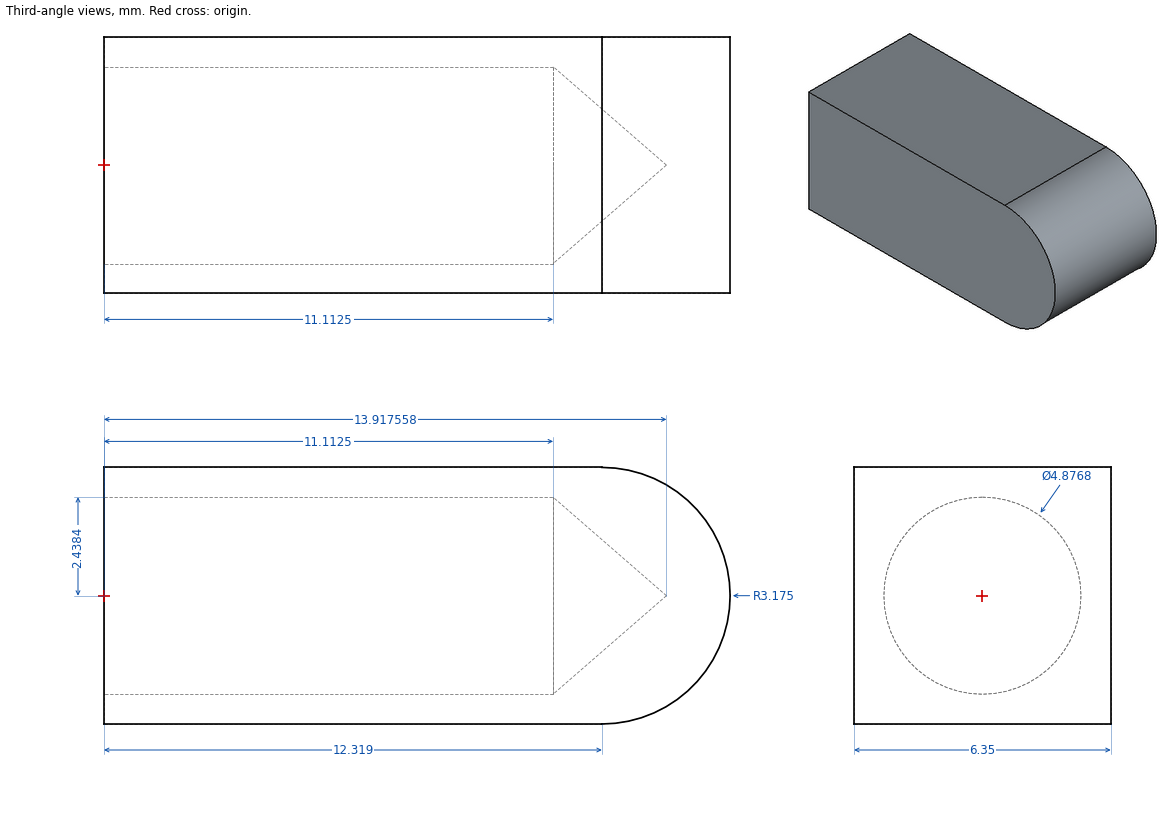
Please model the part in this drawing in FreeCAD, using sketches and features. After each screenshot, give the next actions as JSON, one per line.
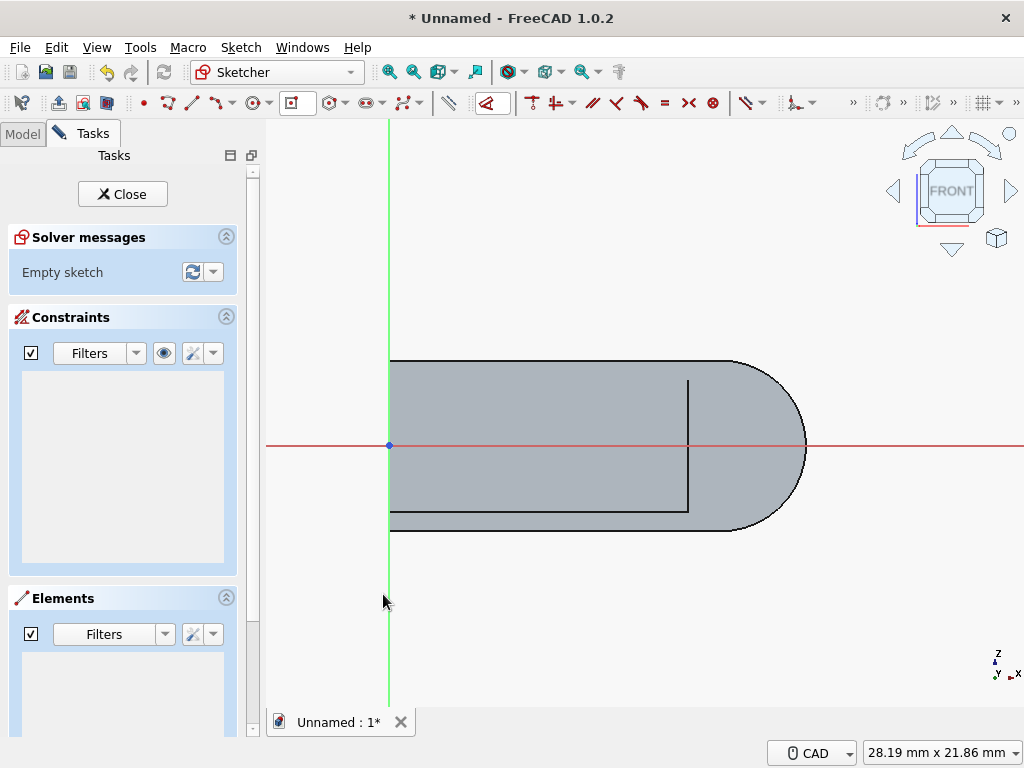
{"action": "key", "text": "g m"}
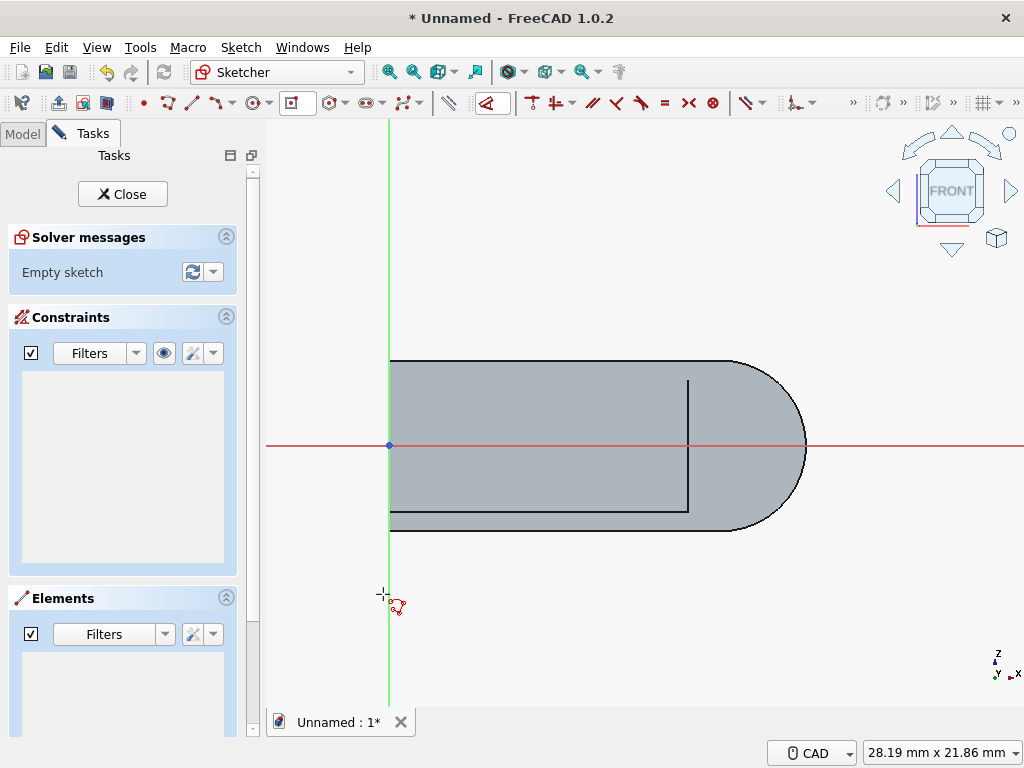
{"action": "left_click", "coordinate": [389, 446]}
{"action": "left_click", "coordinate": [398, 380]}
{"action": "left_click", "coordinate": [688, 380]}
{"action": "left_click", "coordinate": [764, 437]}
{"action": "left_click", "coordinate": [389, 446]}
{"action": "key", "text": "Escape"}
{"action": "key", "text": "Escape"}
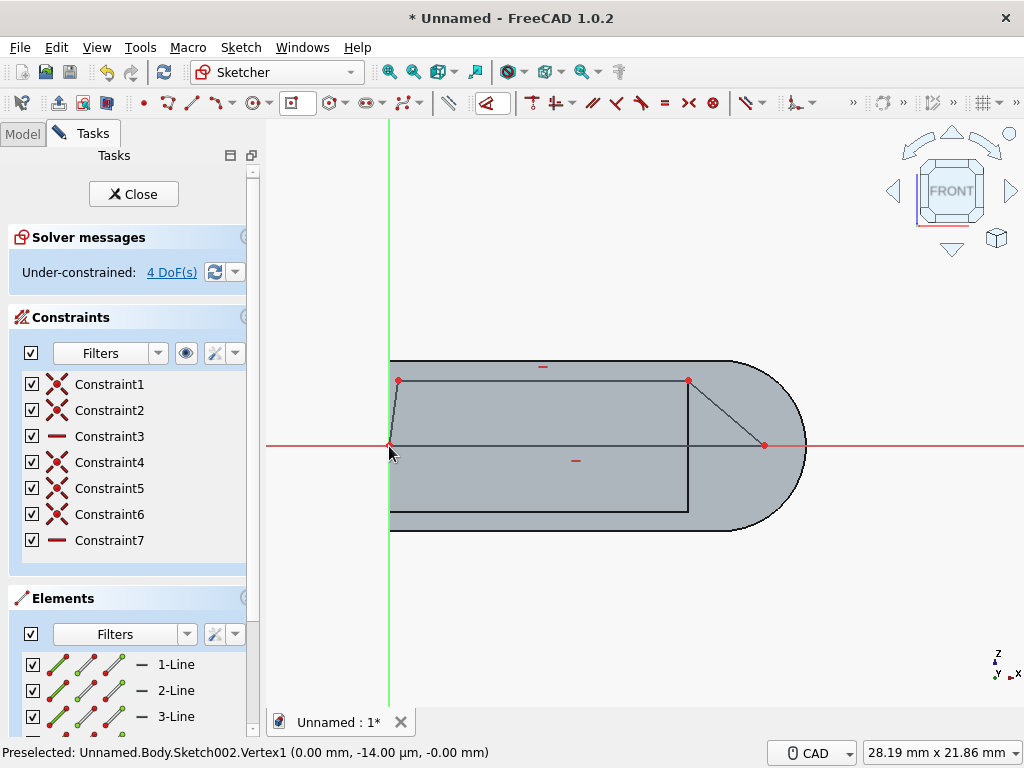
{"action": "left_click", "coordinate": [392, 426]}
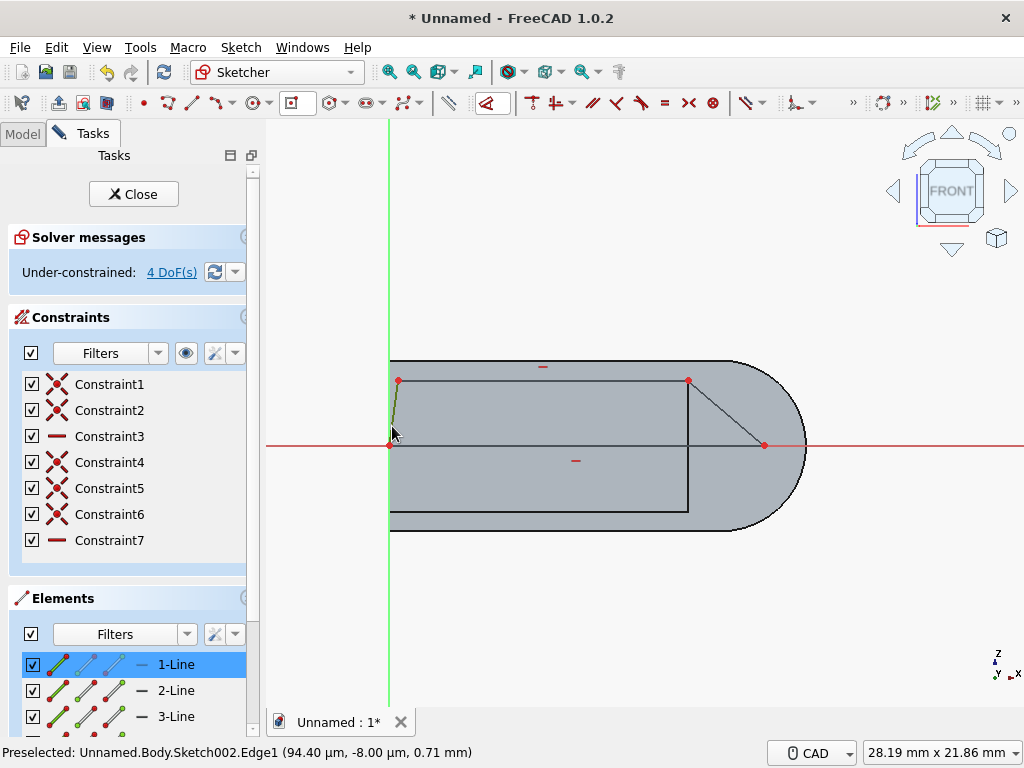
{"action": "key", "text": "v"}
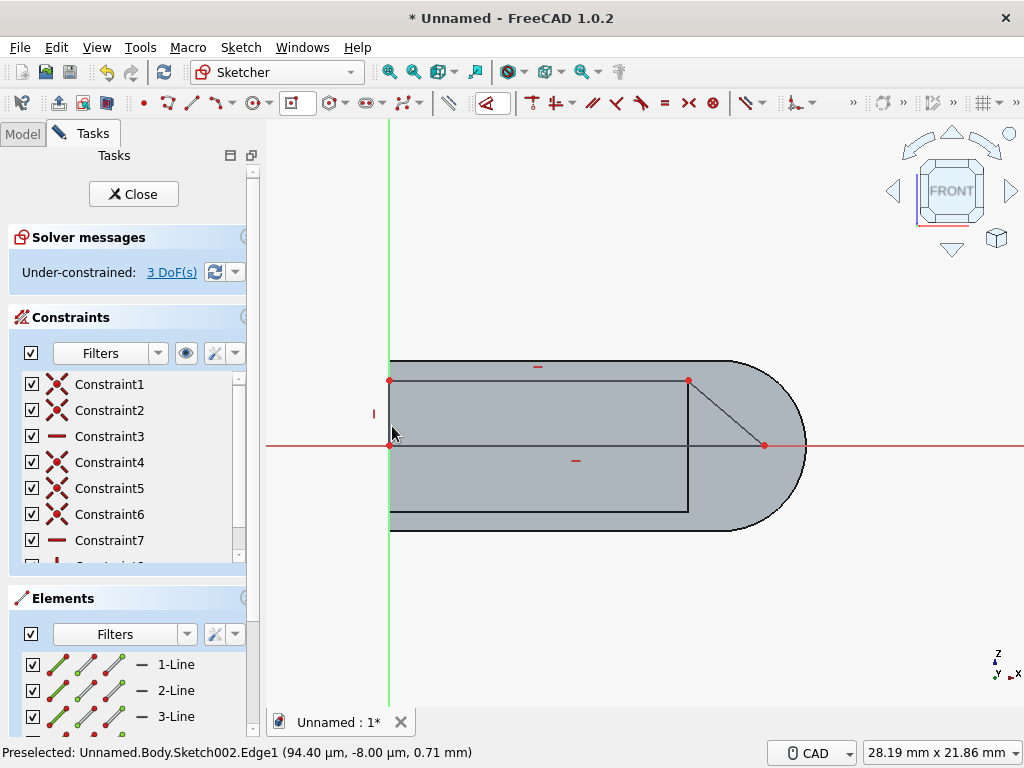
{"action": "left_click", "coordinate": [486, 104]}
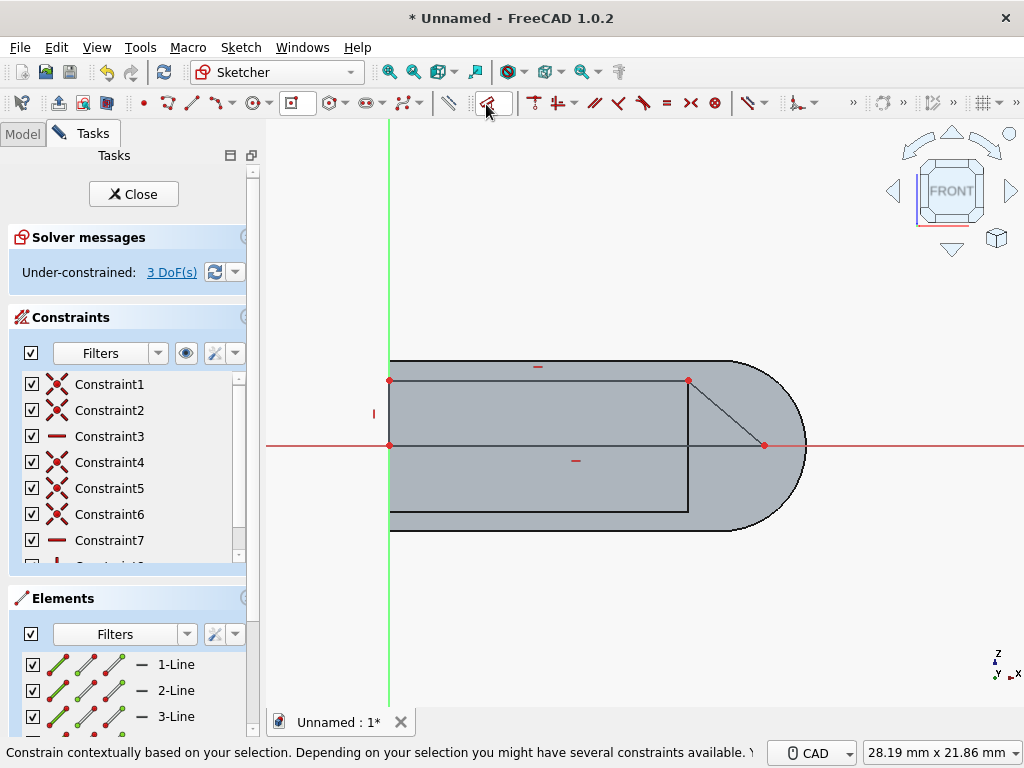
{"action": "left_click", "coordinate": [389, 426]}
{"action": "left_click", "coordinate": [355, 413]}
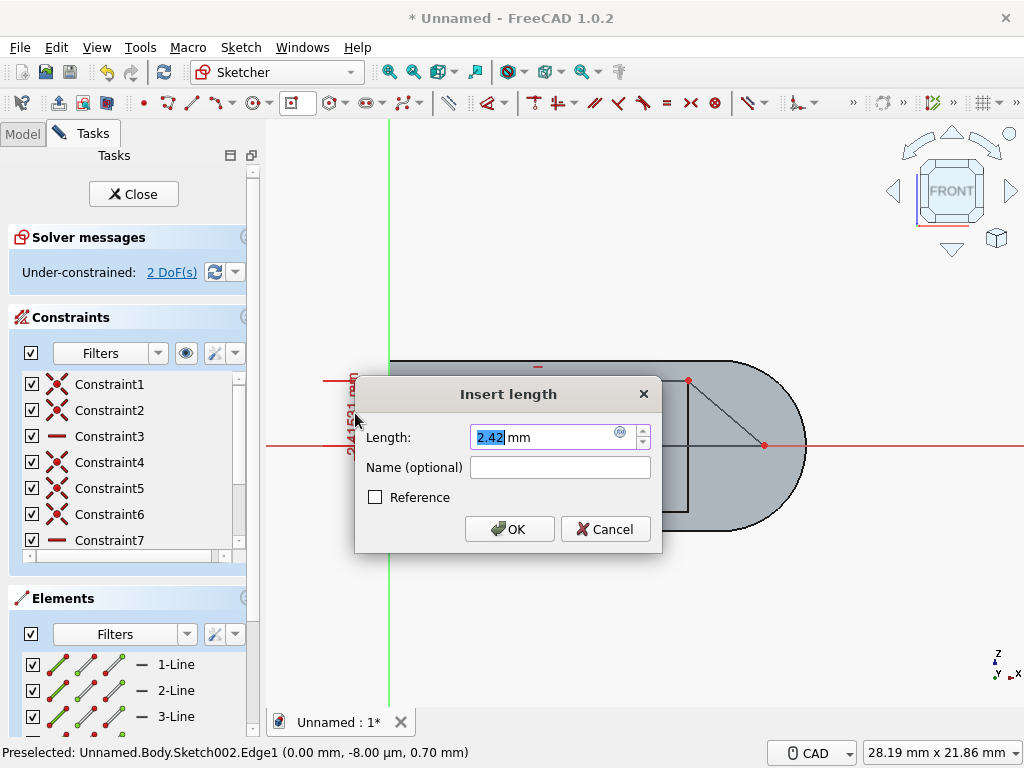
{"action": "type", "text": "2.4384"}
{"action": "key", "text": "Return"}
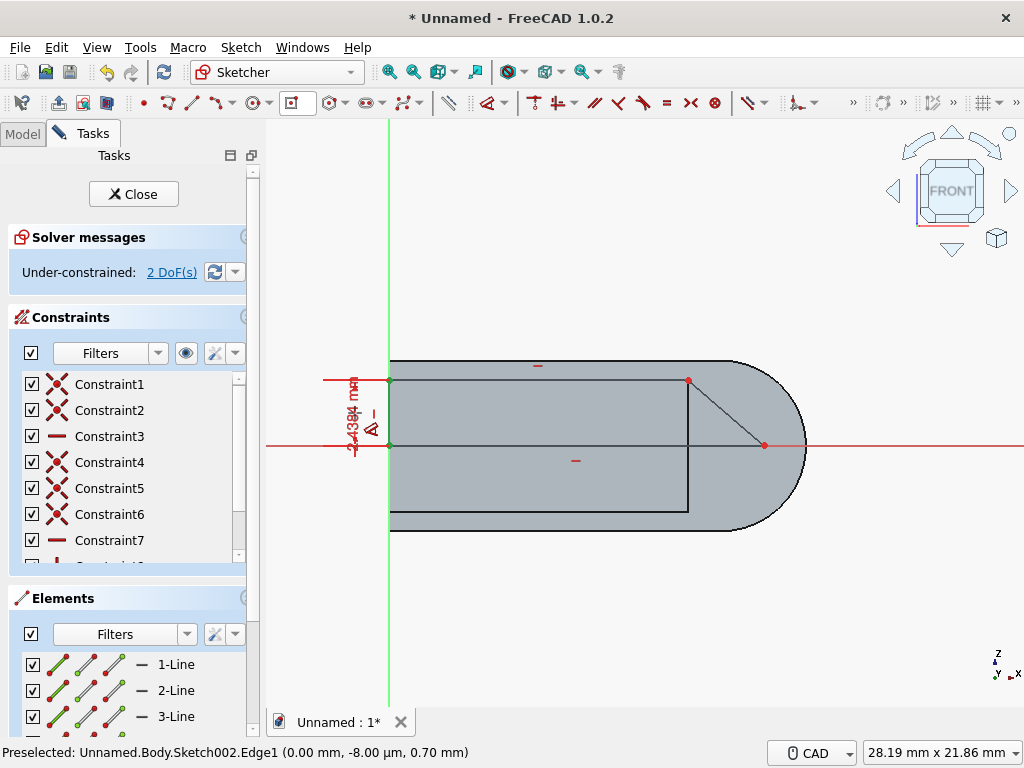
{"action": "left_click", "coordinate": [479, 380]}
{"action": "left_click", "coordinate": [539, 346]}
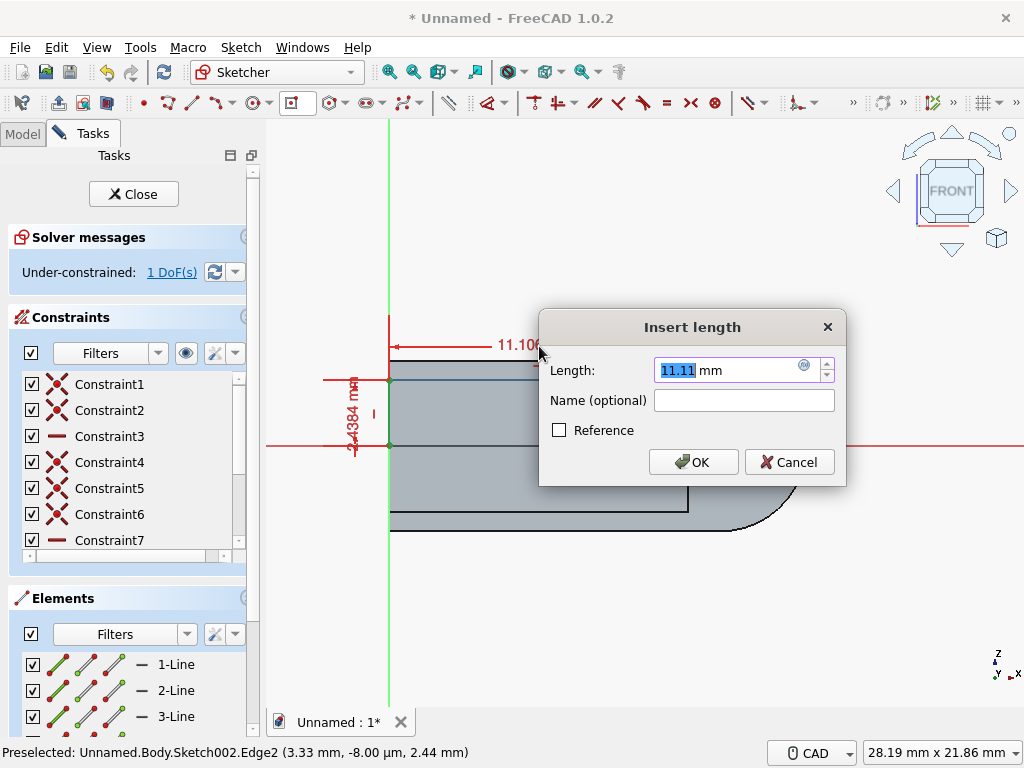
{"action": "type", "text": "11.1125"}
{"action": "key", "text": "Return"}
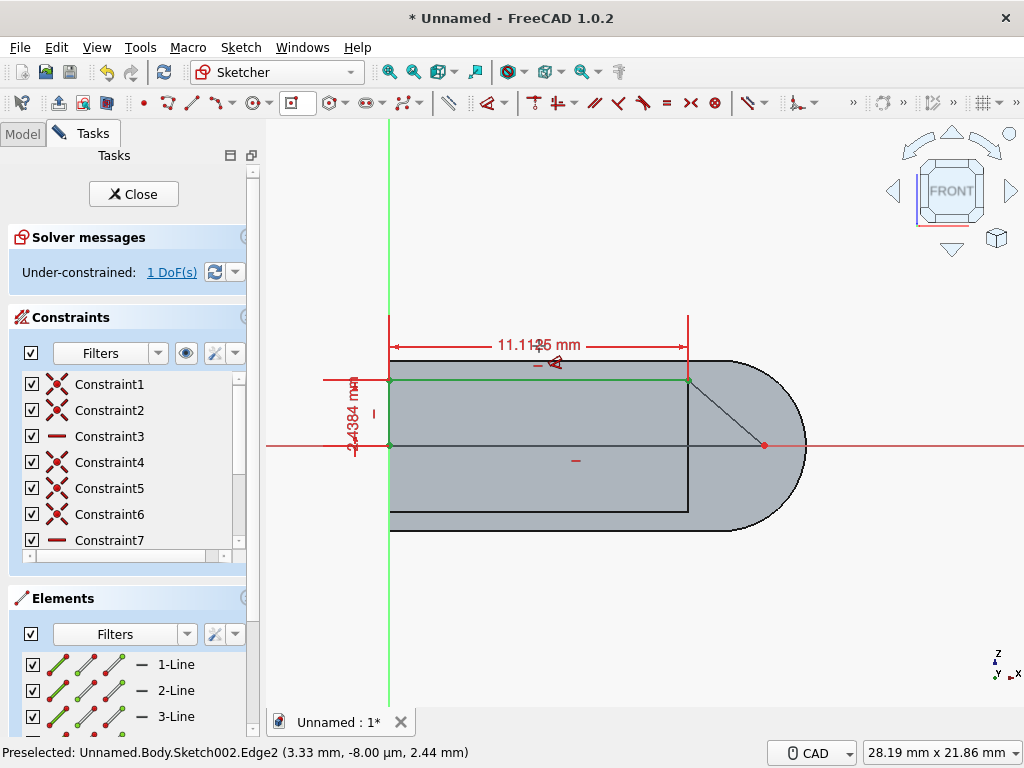
{"action": "left_click", "coordinate": [652, 446]}
{"action": "left_click", "coordinate": [577, 480]}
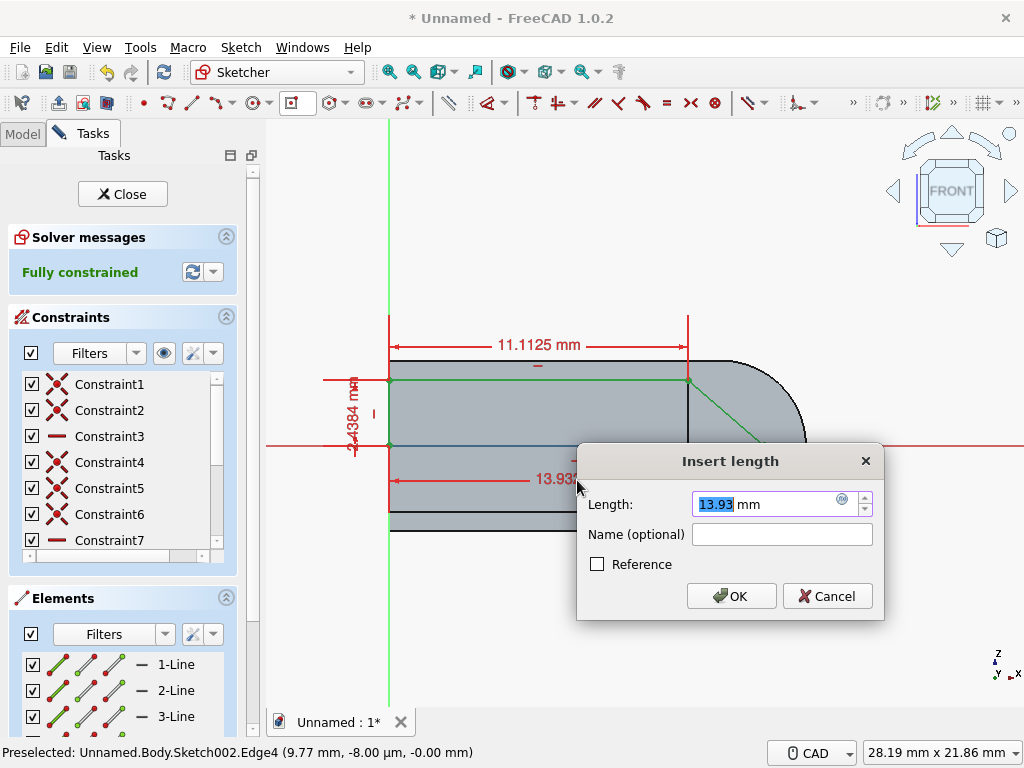
{"action": "type", "text": "13.917558"}
{"action": "key", "text": "Return"}
{"action": "key", "text": "Escape"}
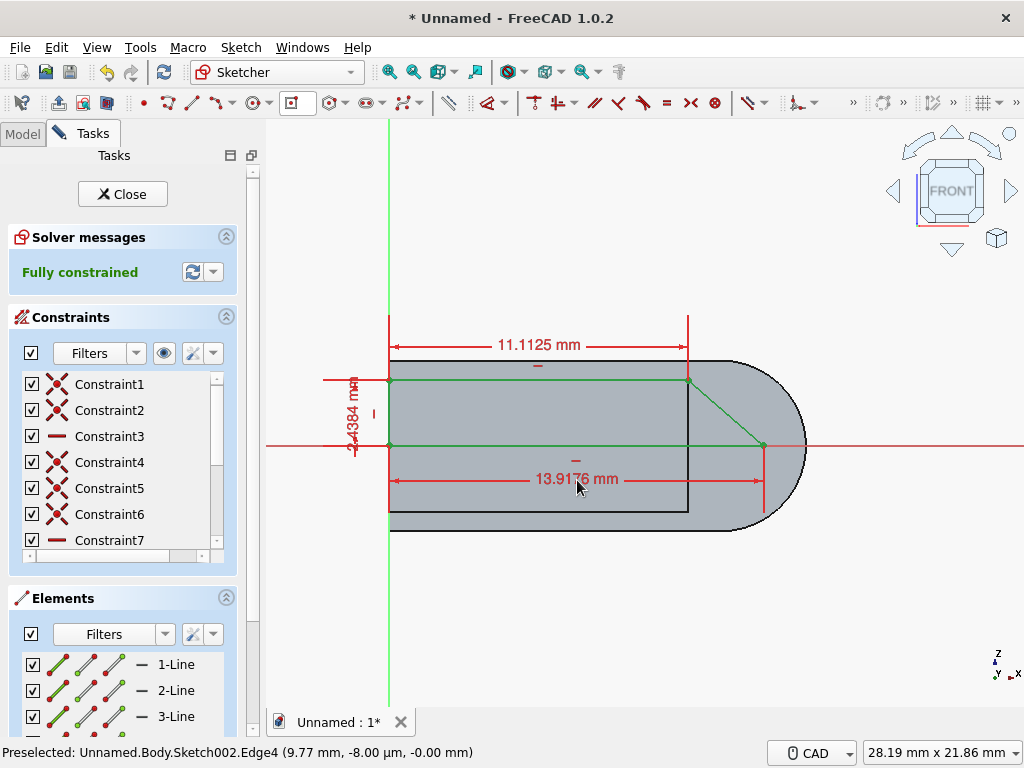
{"action": "left_click", "coordinate": [123, 194]}